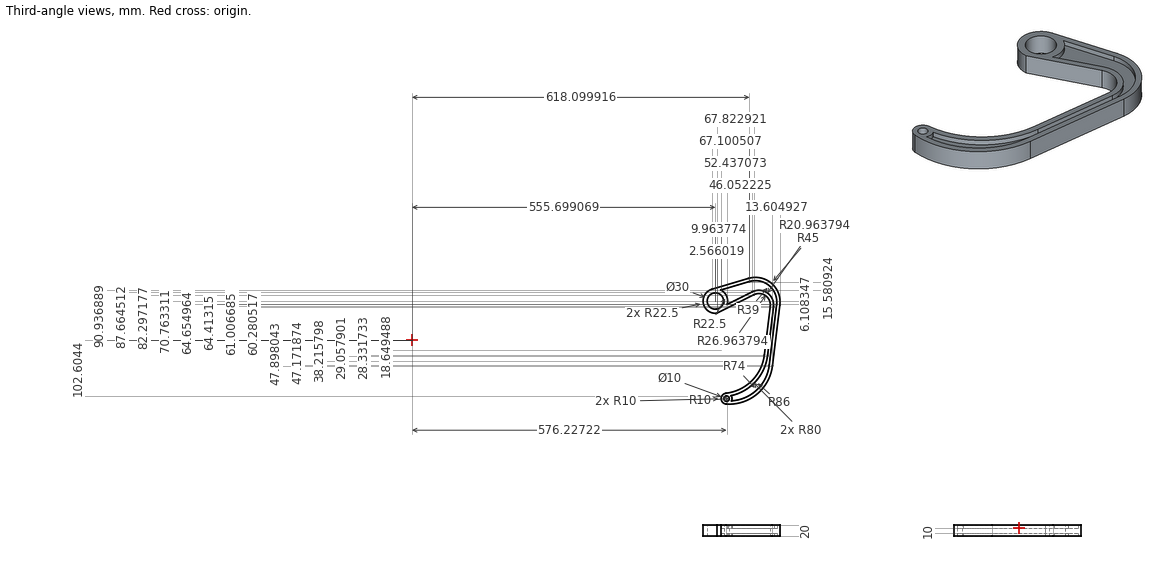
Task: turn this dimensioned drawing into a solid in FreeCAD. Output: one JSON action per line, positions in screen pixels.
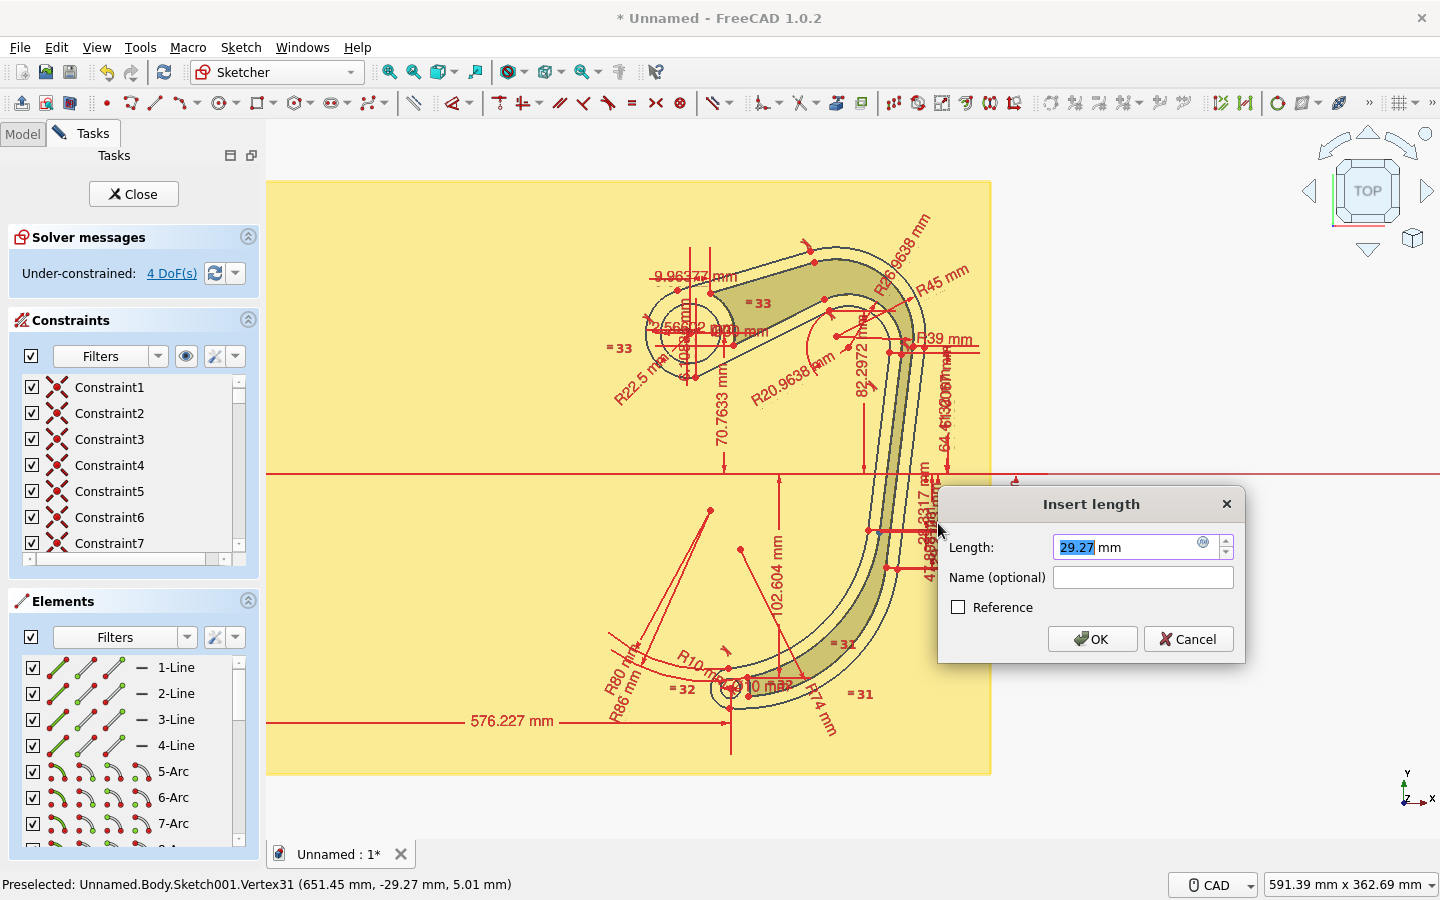
{"action": "type", "text": "29.057901"}
{"action": "key", "text": "Return"}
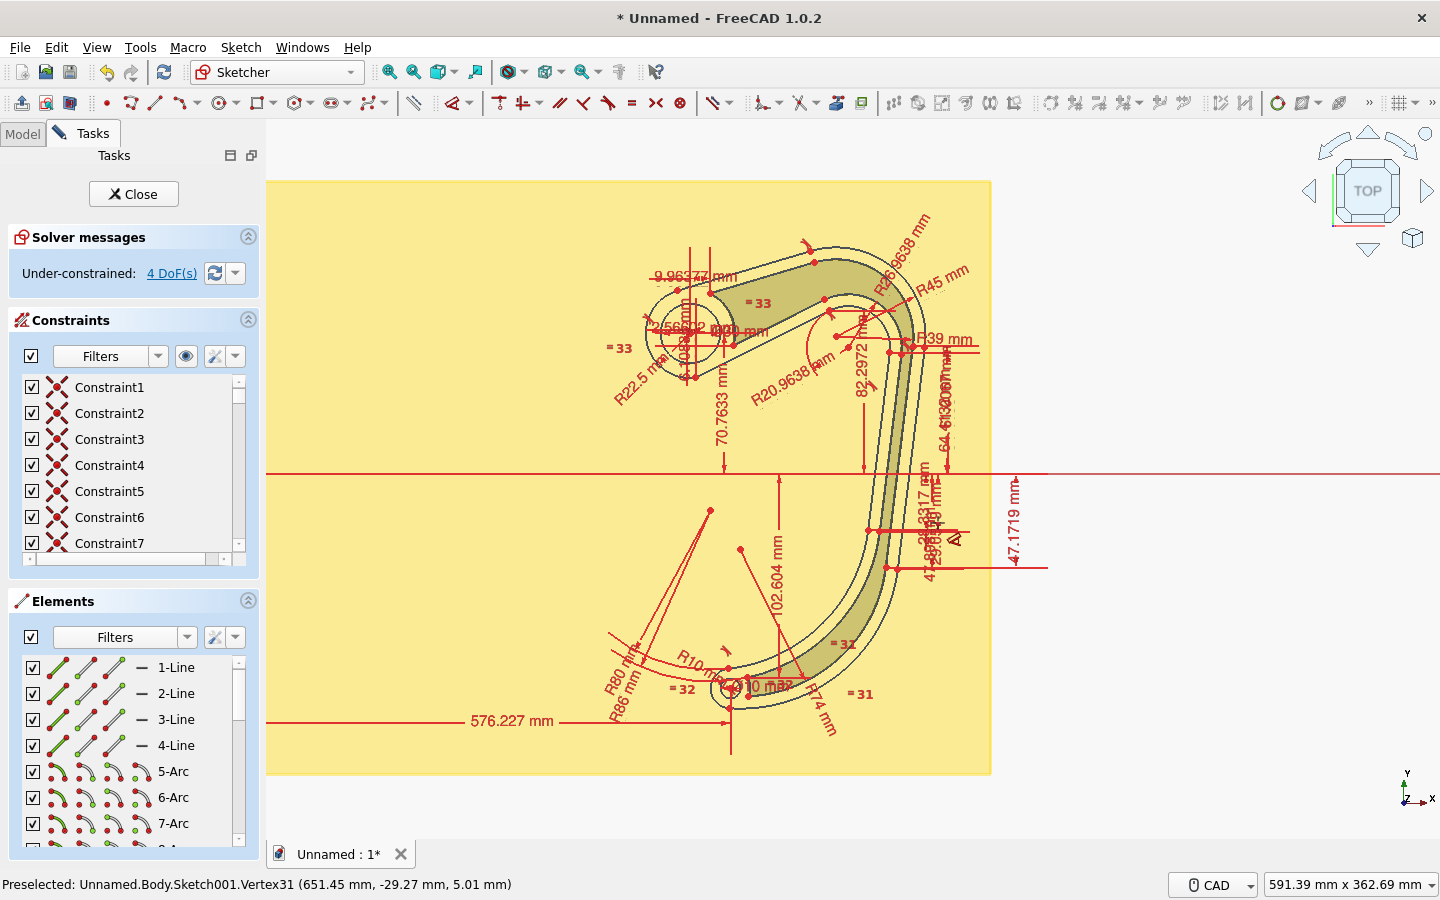
{"action": "left_click", "coordinate": [771, 263]}
{"action": "left_click", "coordinate": [744, 217]}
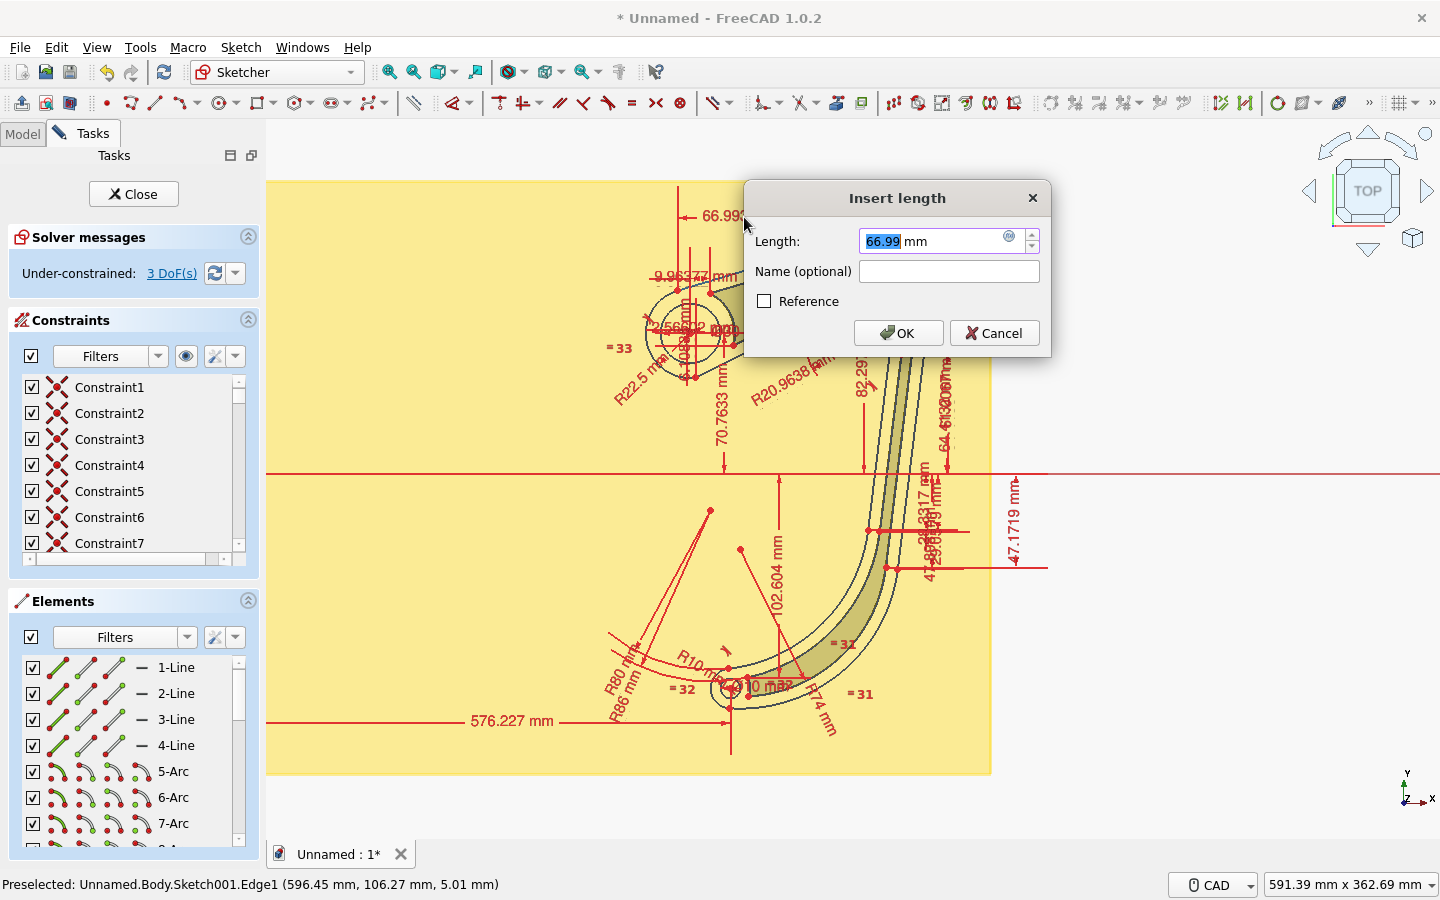
{"action": "type", "text": "67.100507"}
{"action": "key", "text": "Return"}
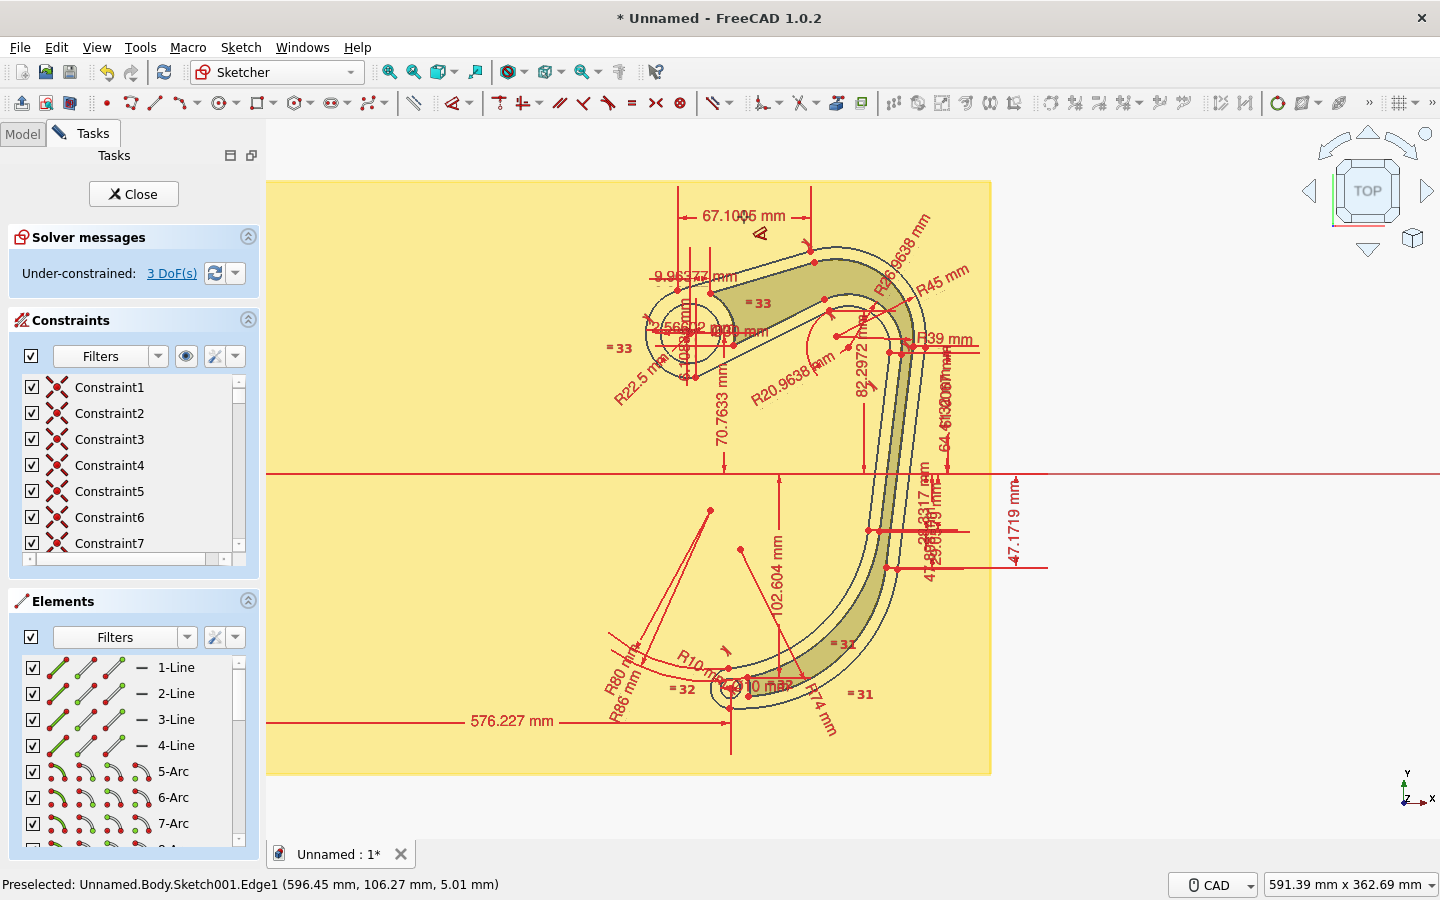
{"action": "left_click", "coordinate": [736, 358]}
{"action": "left_click", "coordinate": [810, 412]}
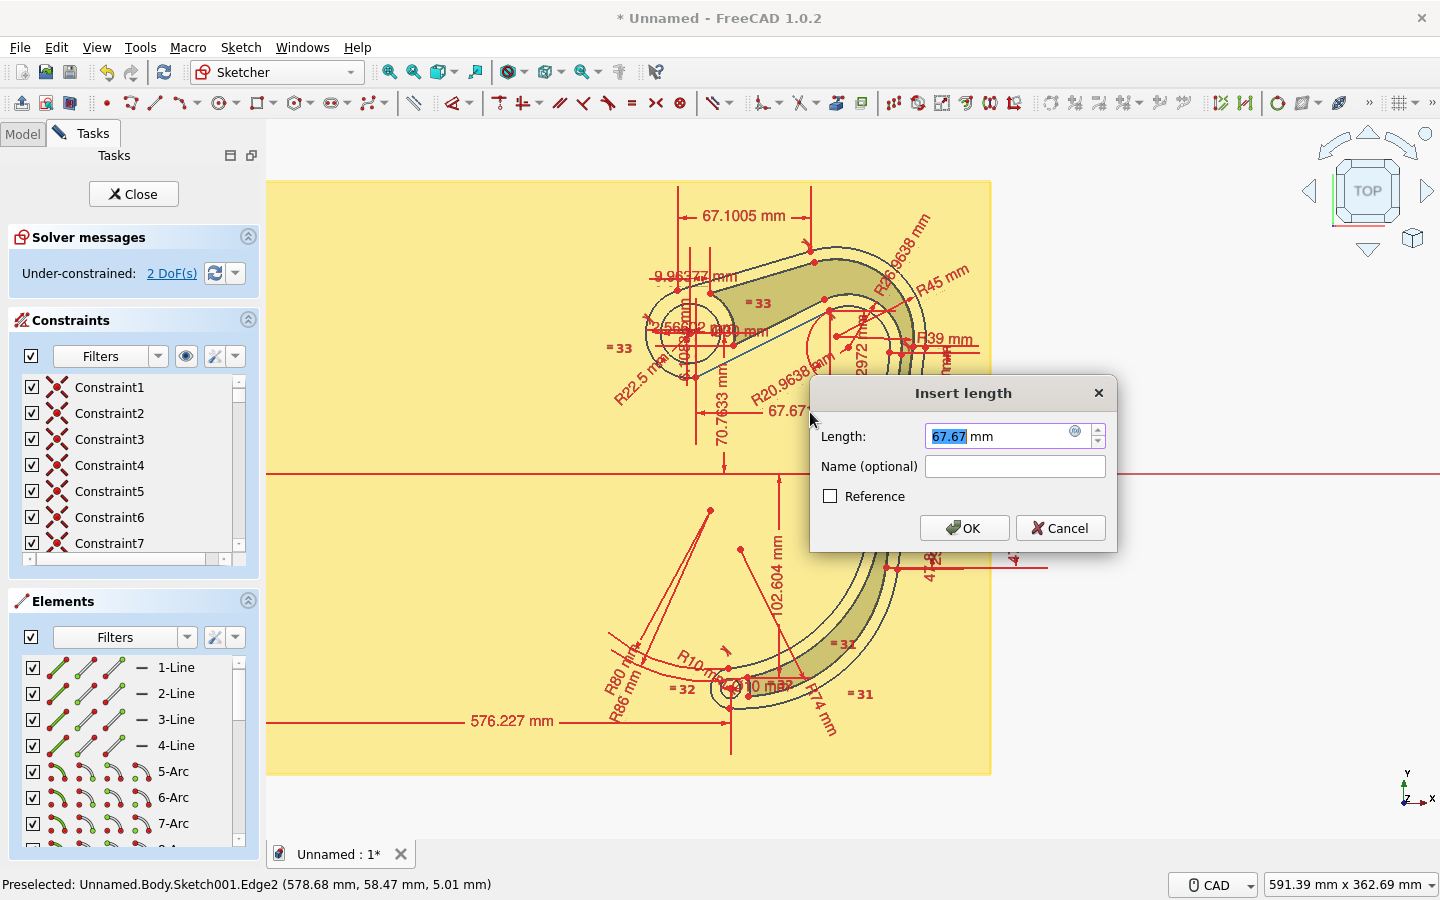
{"action": "type", "text": "67.822921"}
{"action": "key", "text": "Return"}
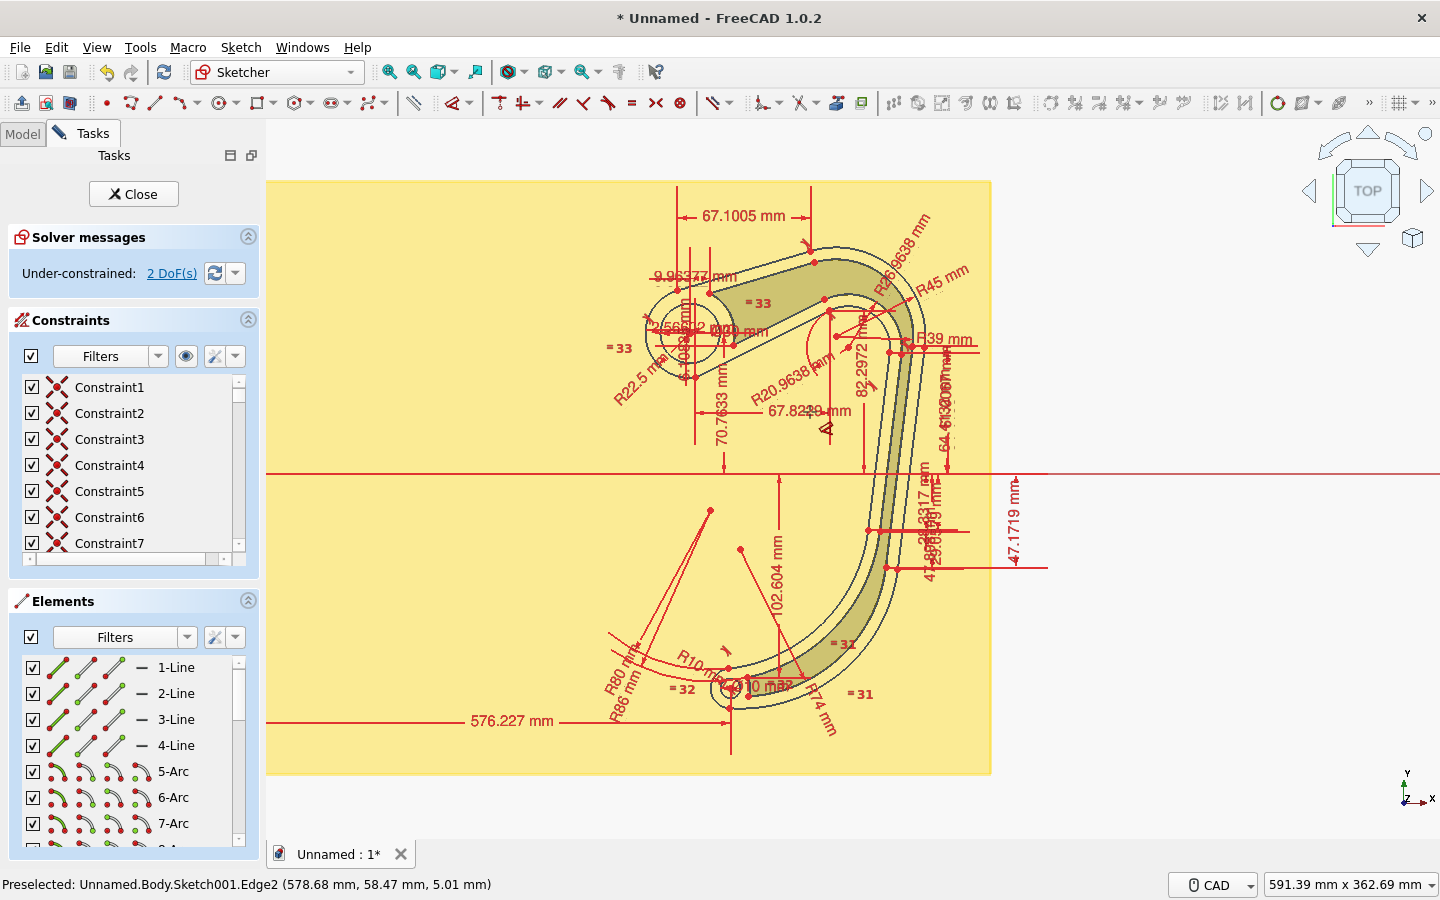
{"action": "scroll", "coordinate": [906, 503], "scroll_direction": "up", "scroll_amount": 2}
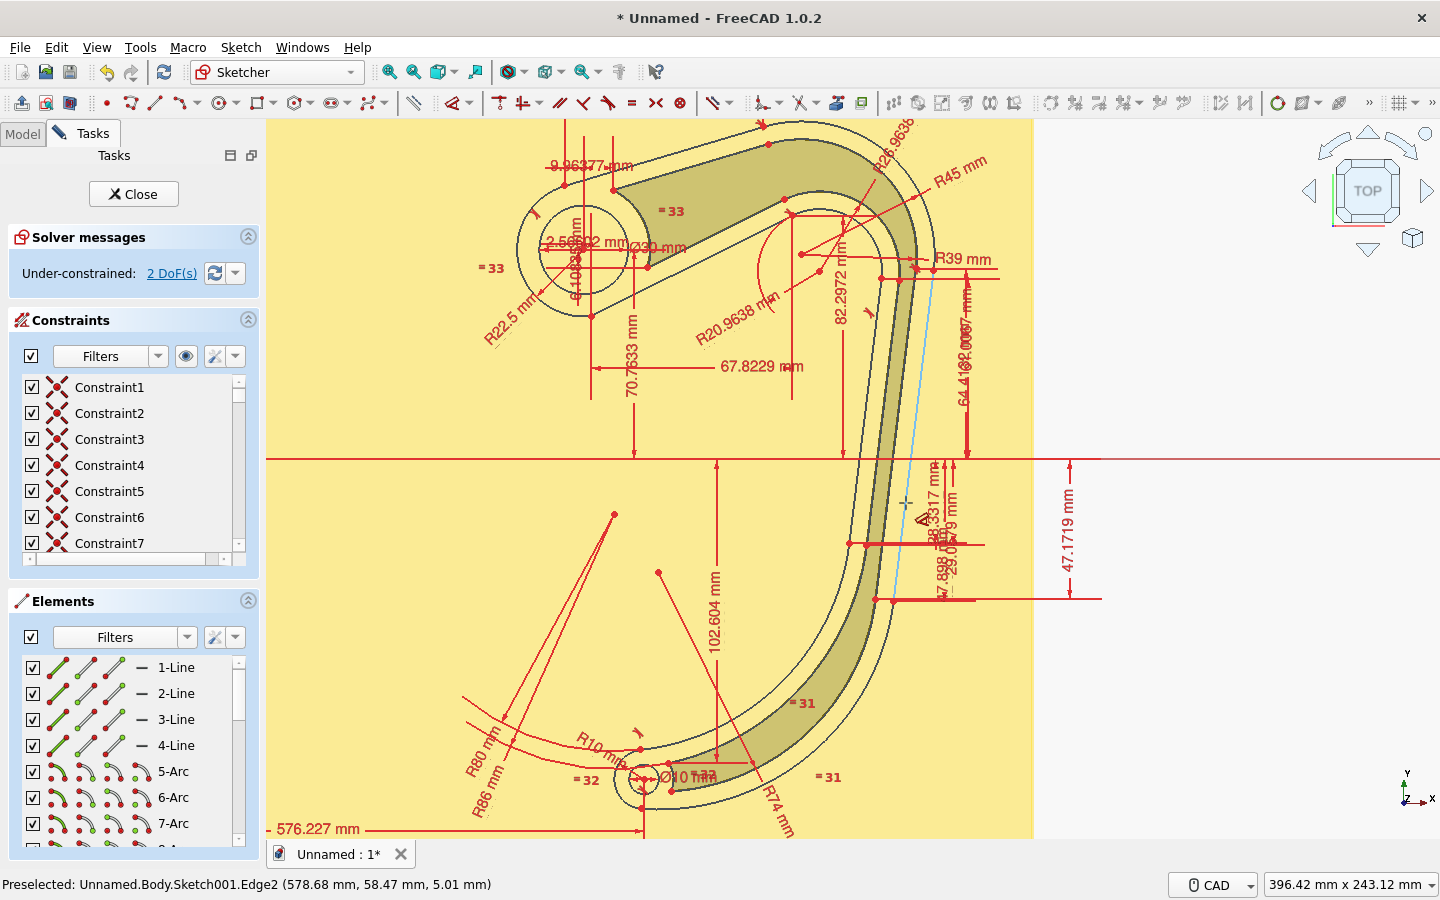
{"action": "left_click", "coordinate": [906, 502]}
{"action": "left_click", "coordinate": [914, 635]}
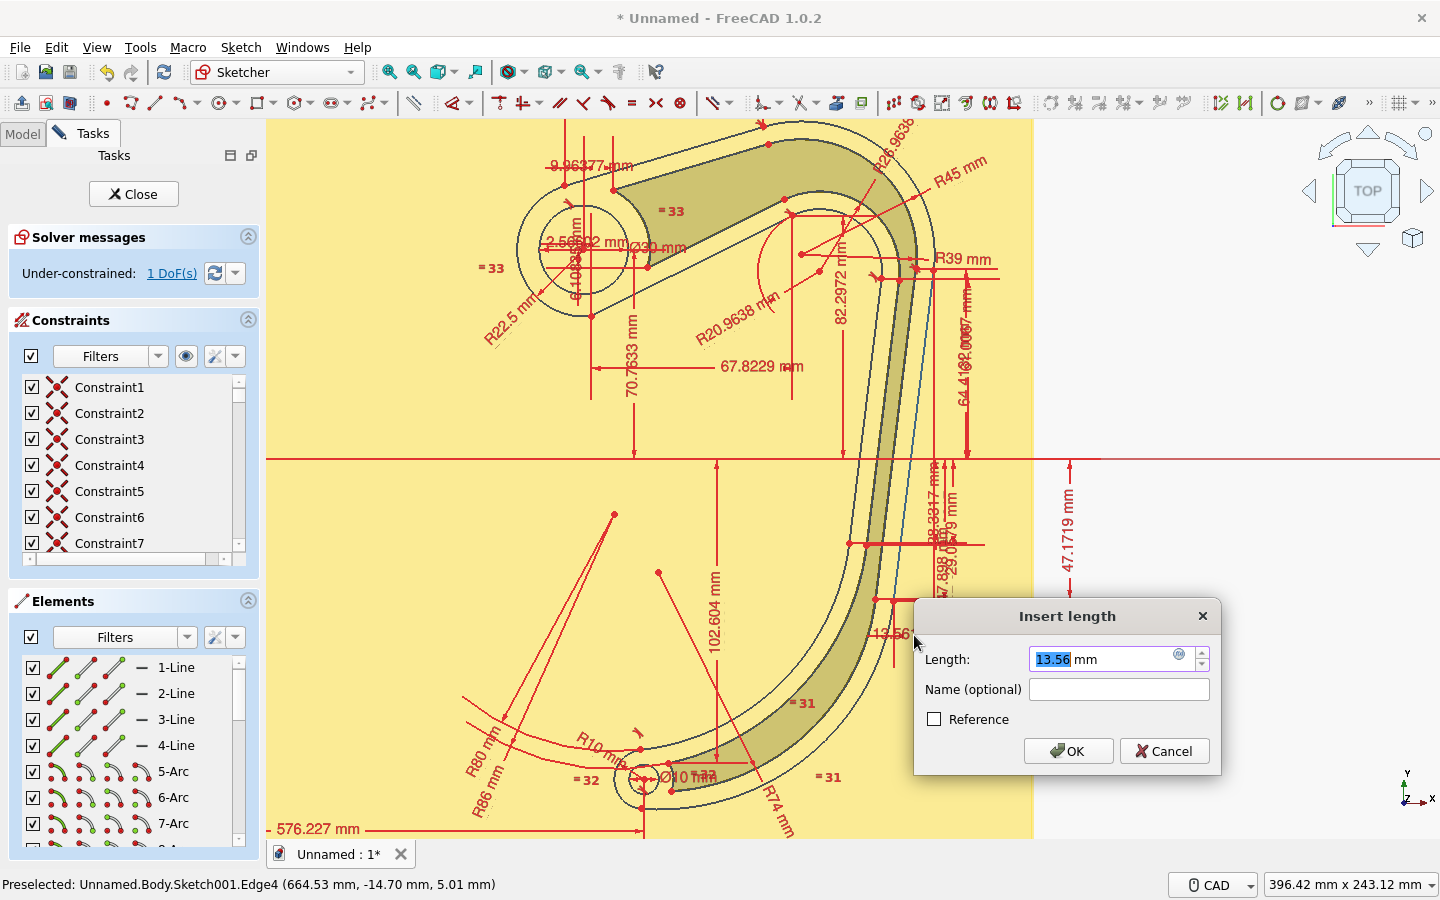
{"action": "type", "text": "13.604927"}
{"action": "key", "text": "Return"}